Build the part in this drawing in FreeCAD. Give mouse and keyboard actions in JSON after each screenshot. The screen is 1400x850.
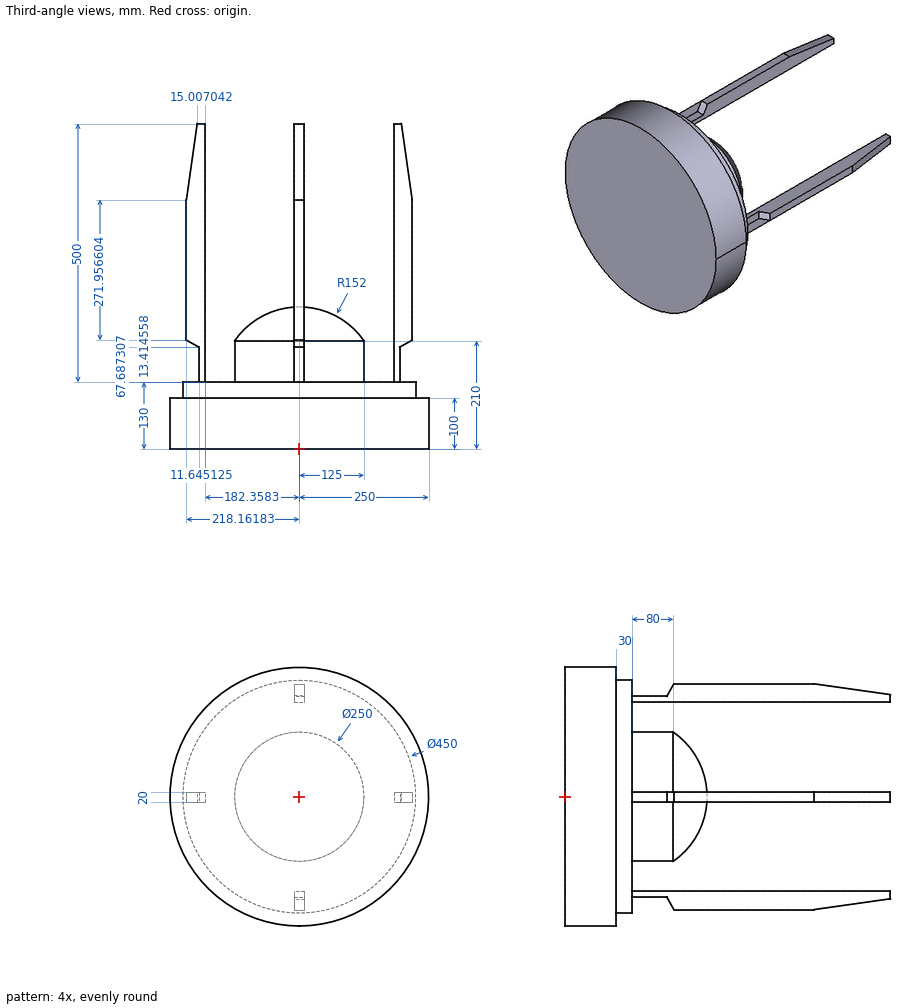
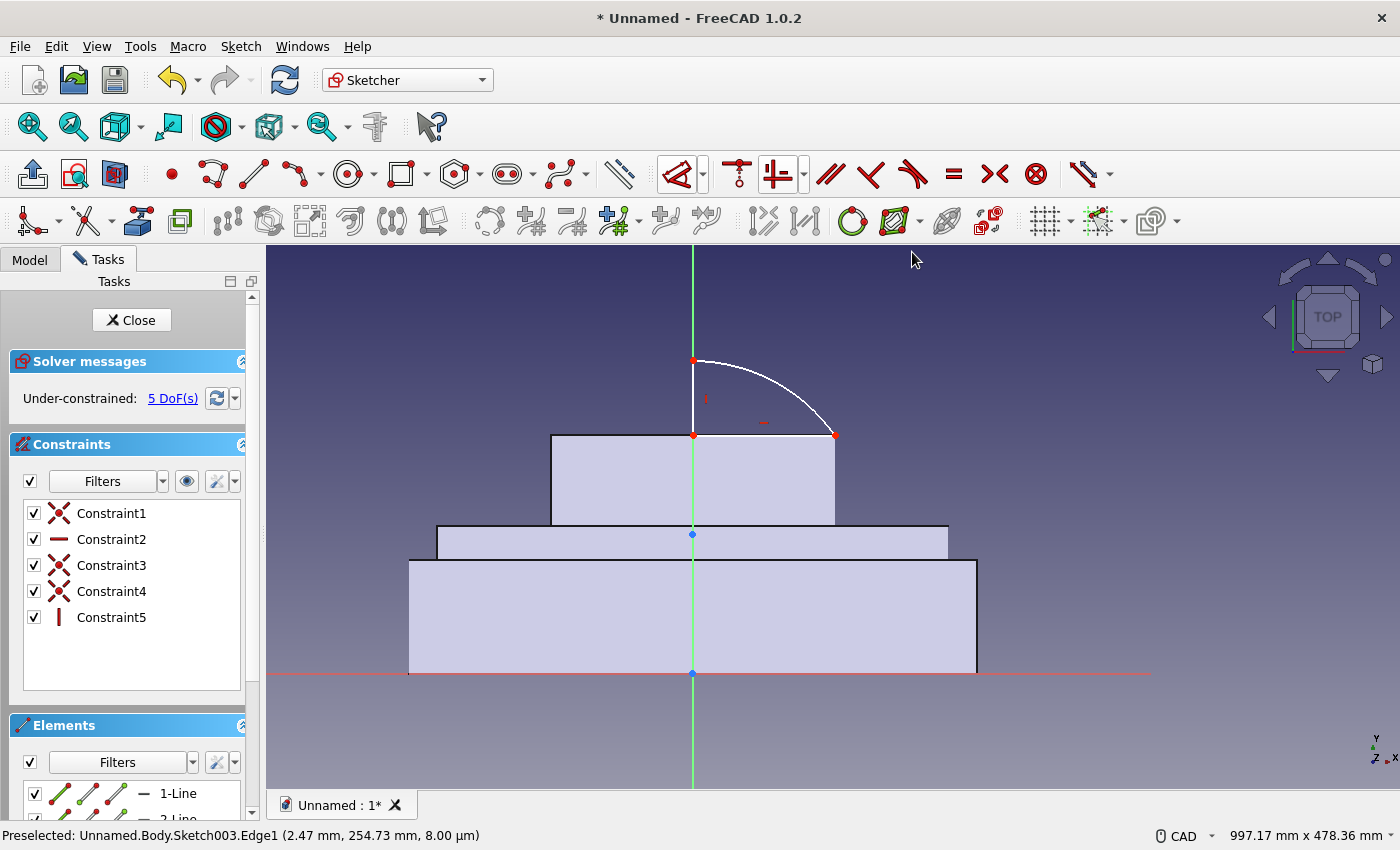
{"action": "left_click", "coordinate": [692, 535]}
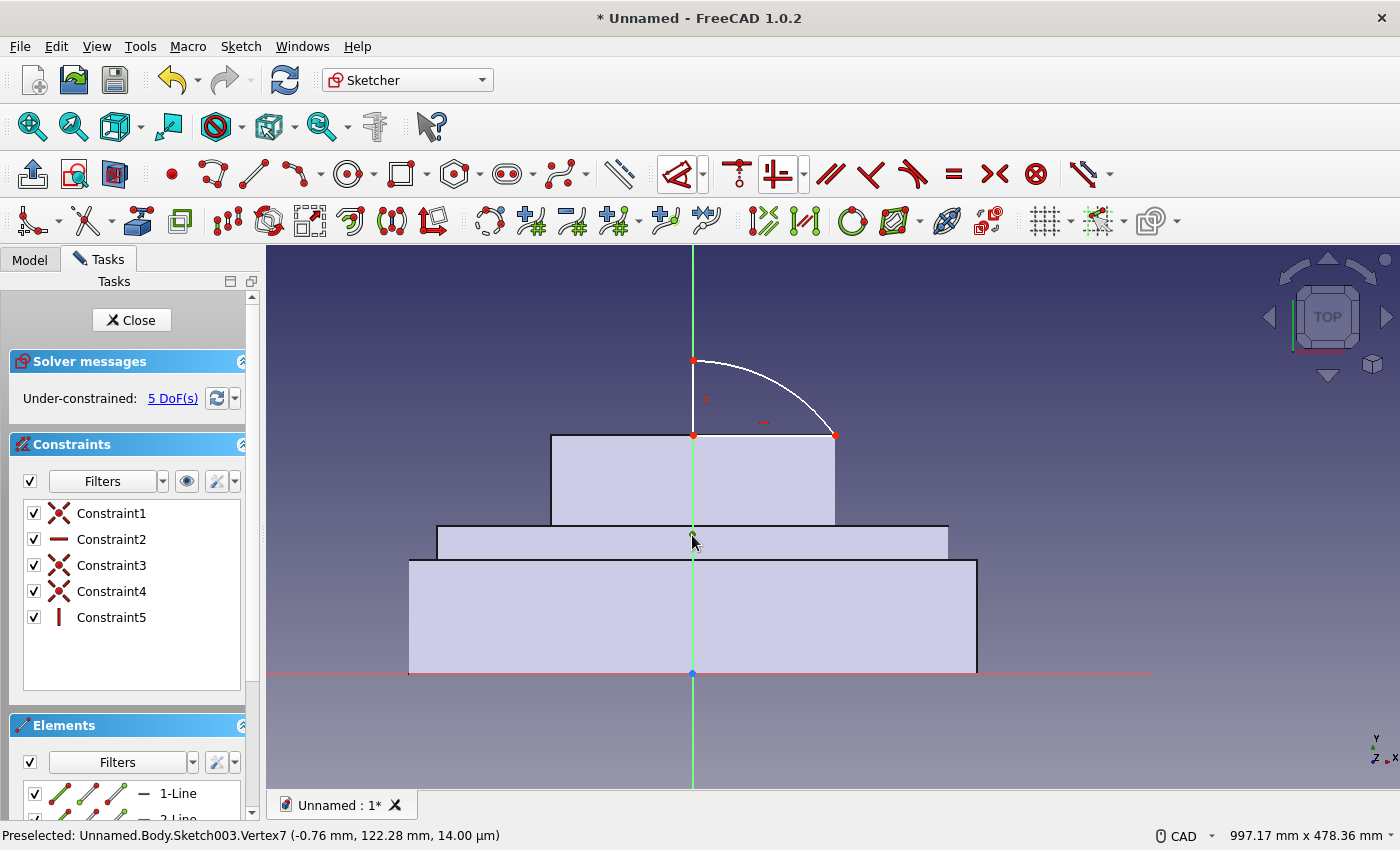
{"action": "left_click", "coordinate": [693, 726]}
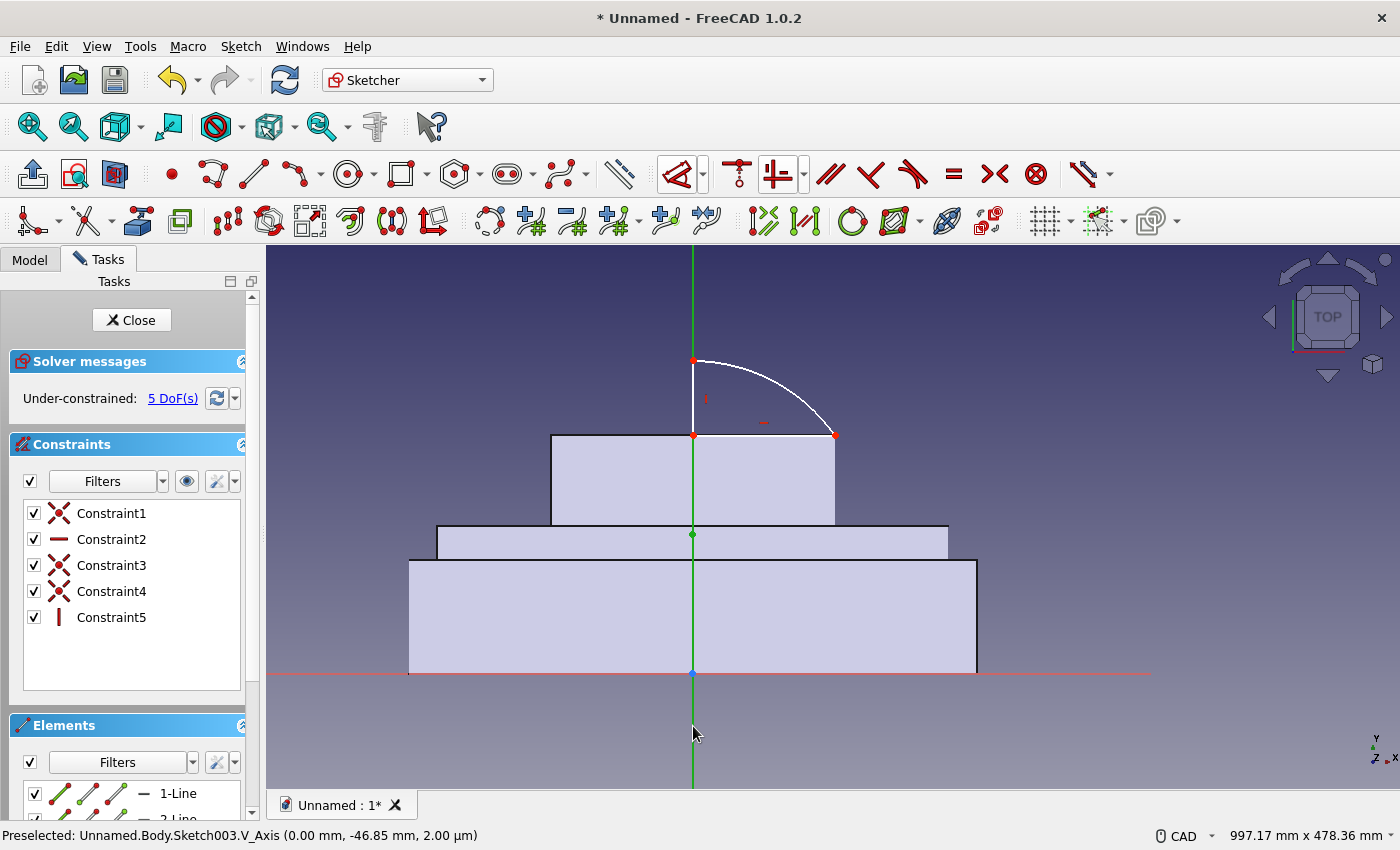
{"action": "left_click", "coordinate": [737, 174]}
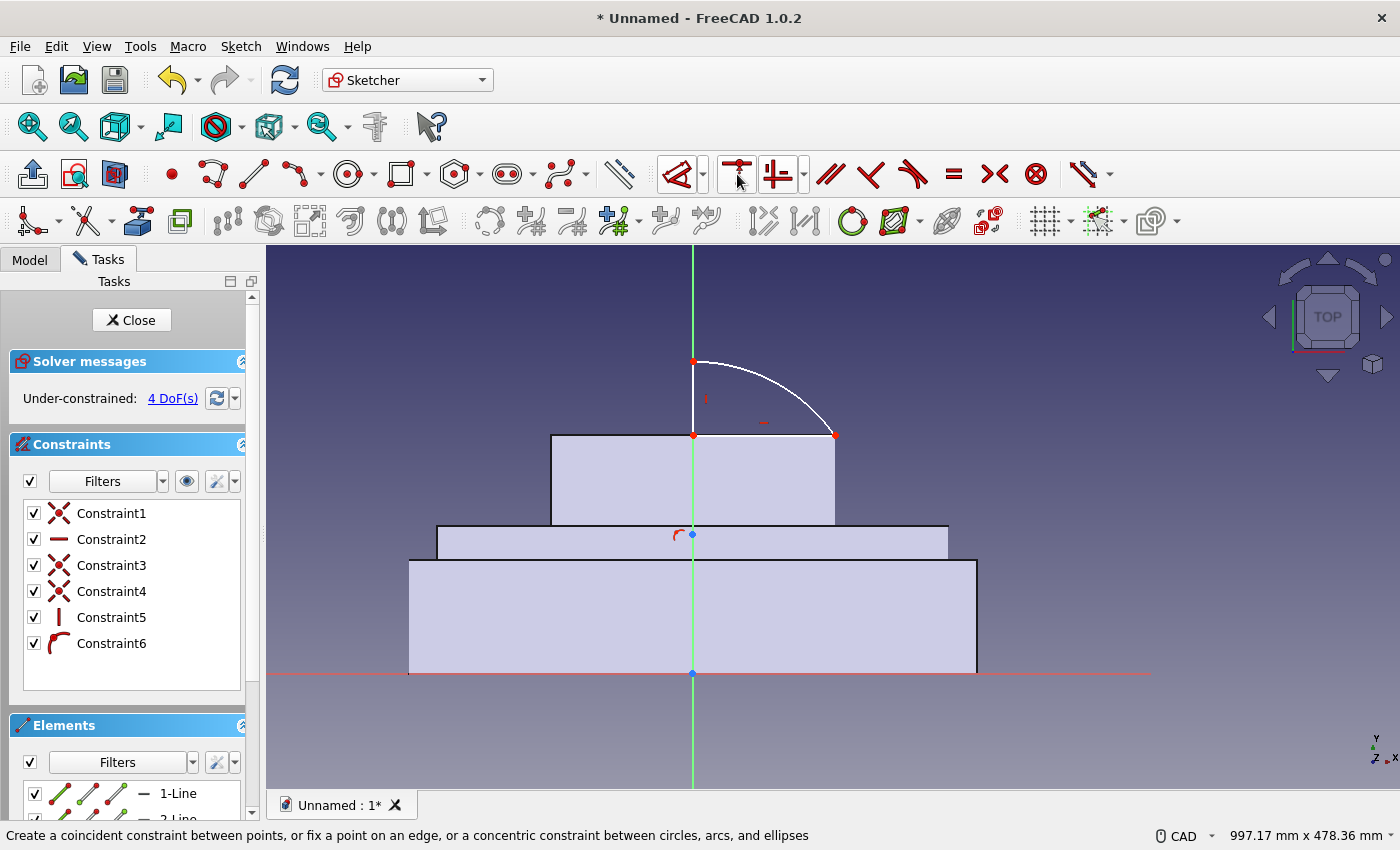
{"action": "left_click", "coordinate": [801, 400]}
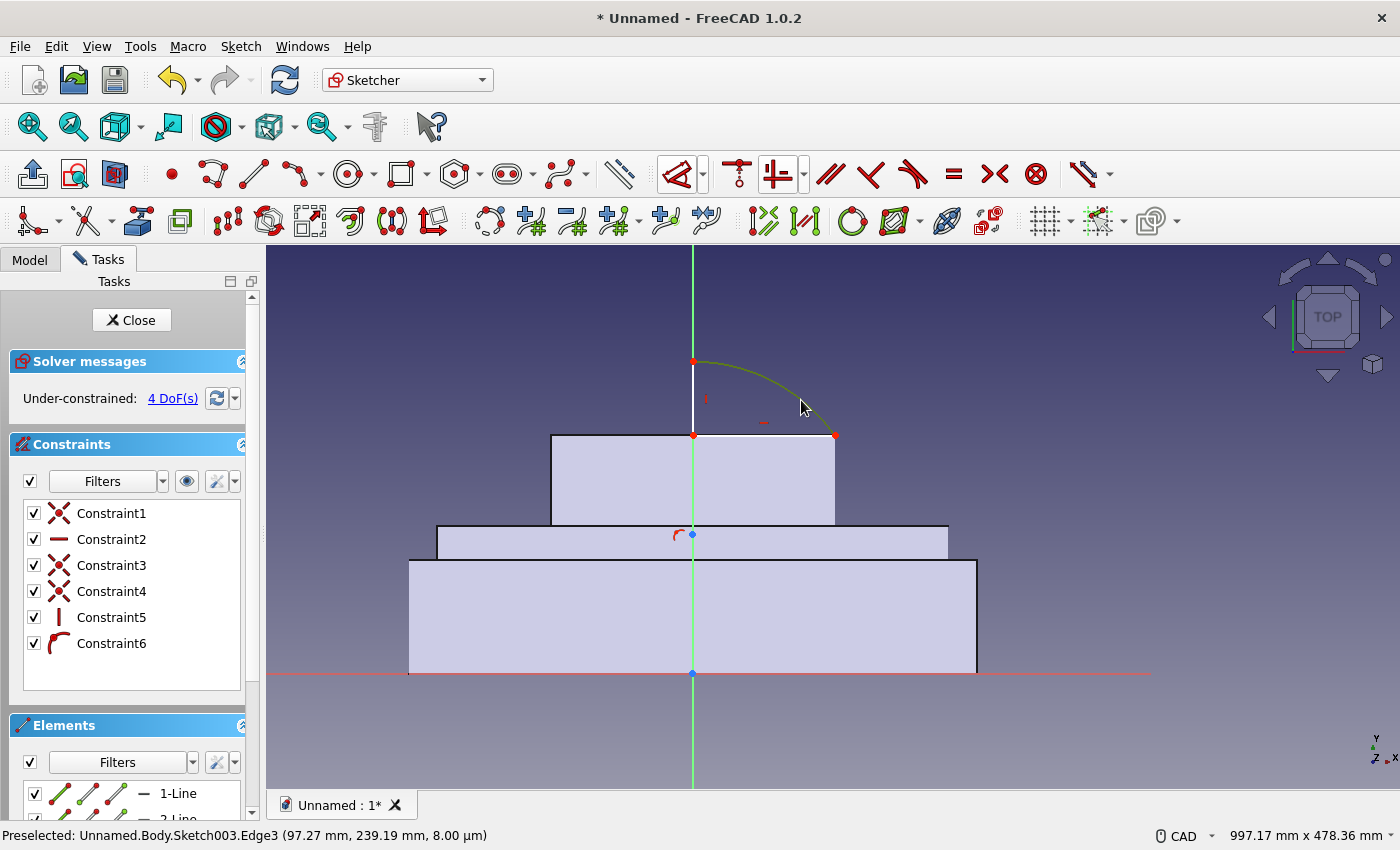
{"action": "key", "text": "k r"}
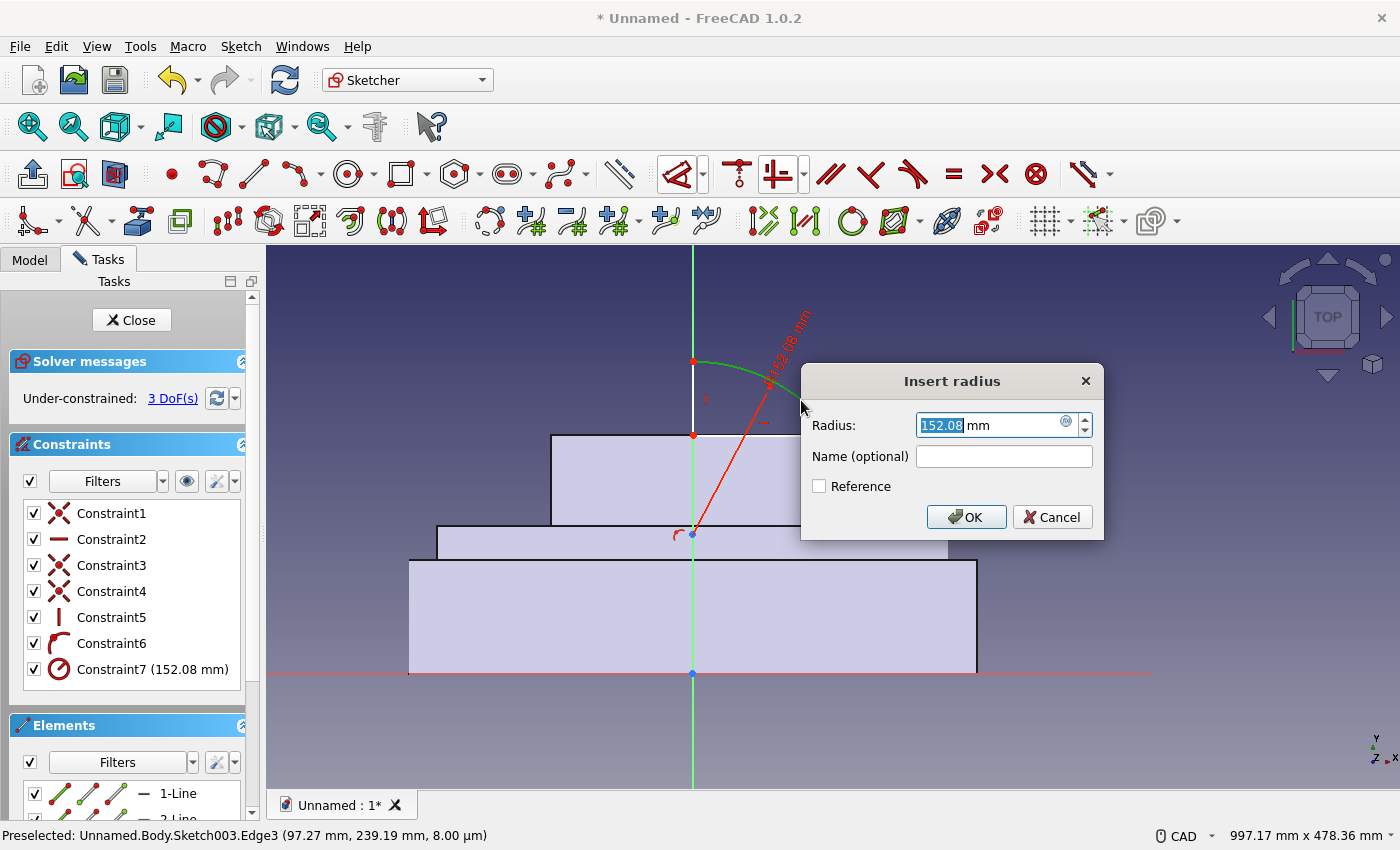
{"action": "type", "text": "152"}
{"action": "key", "text": "Return"}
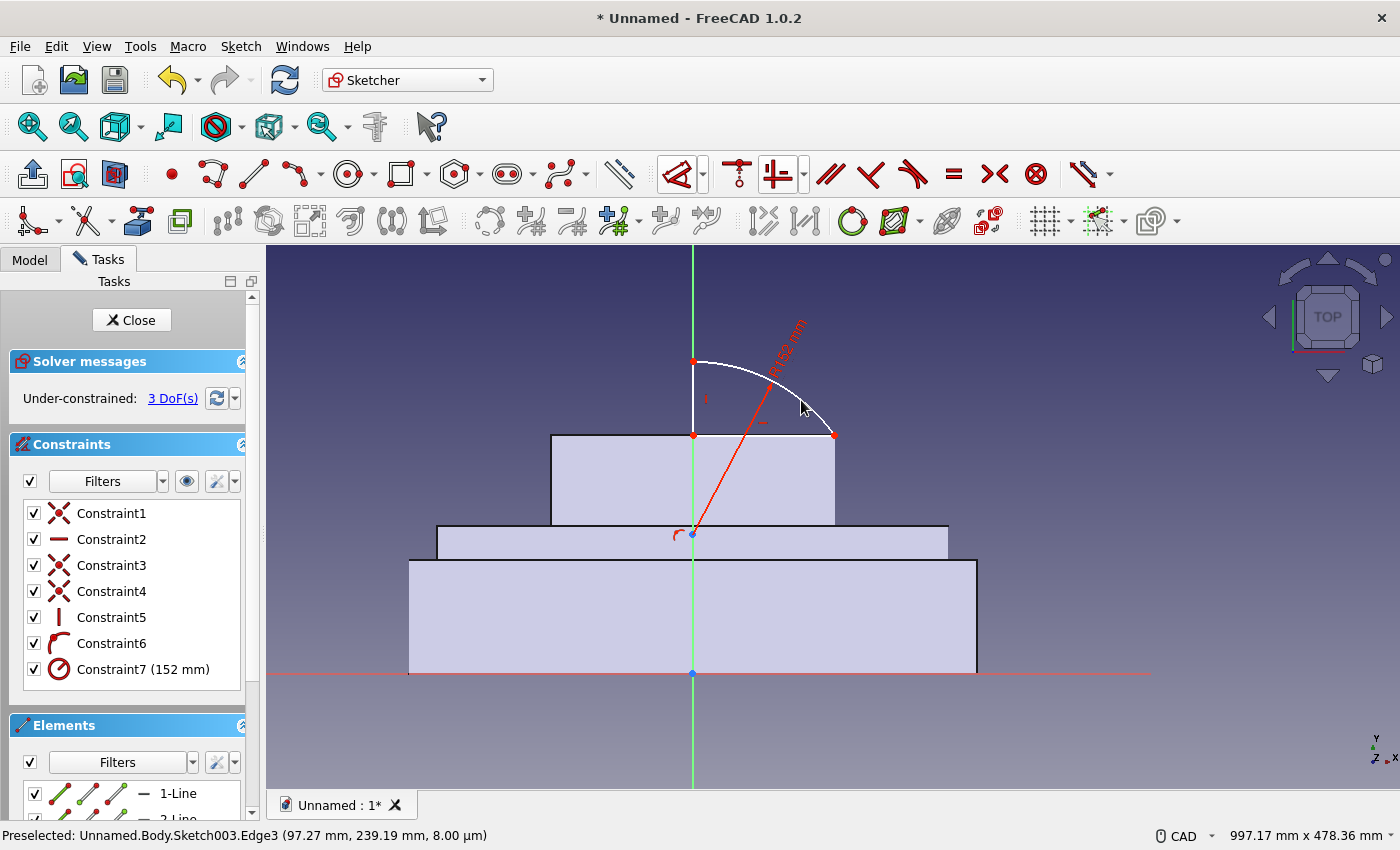
{"action": "left_click", "coordinate": [693, 362]}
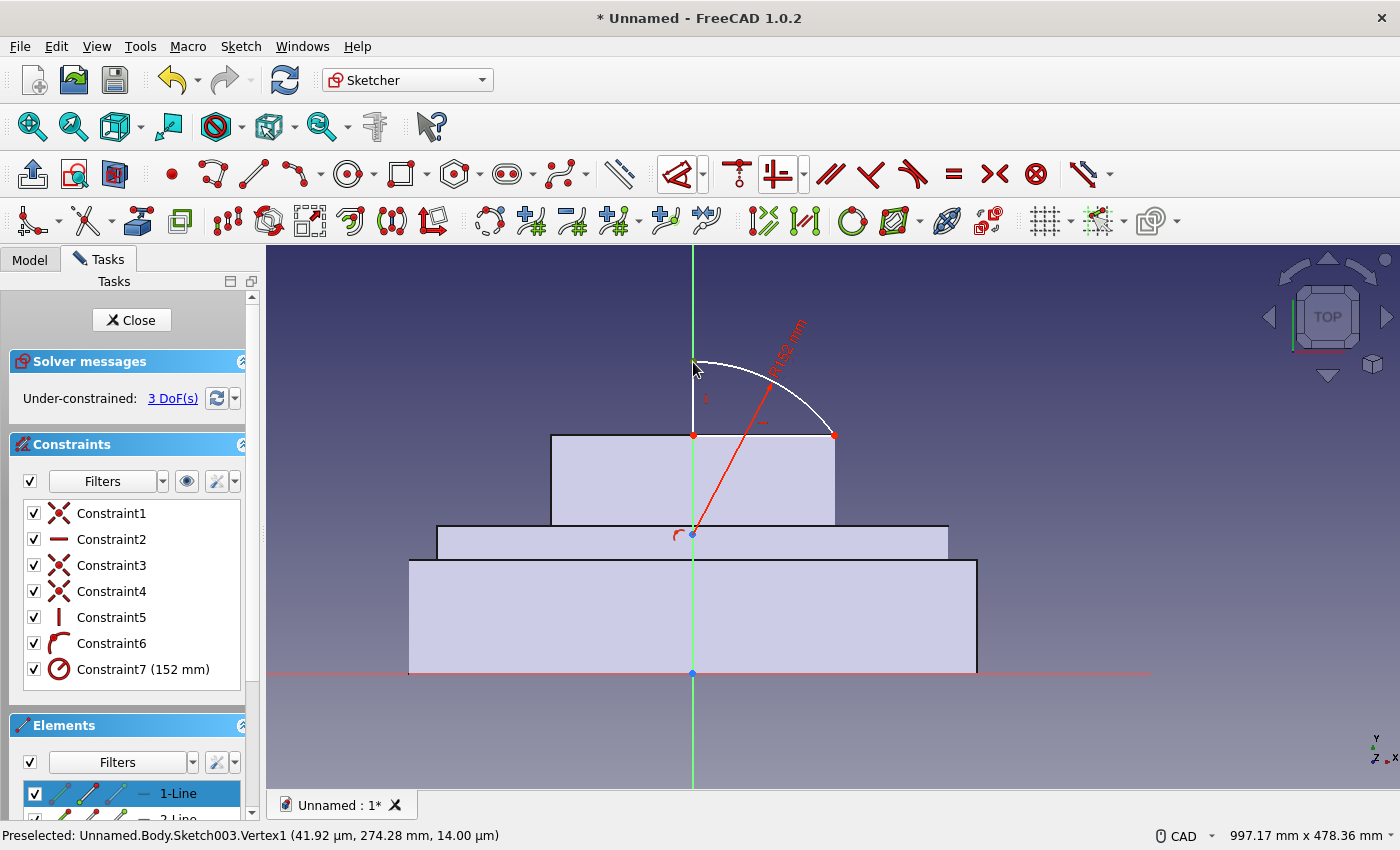
{"action": "left_click", "coordinate": [693, 726]}